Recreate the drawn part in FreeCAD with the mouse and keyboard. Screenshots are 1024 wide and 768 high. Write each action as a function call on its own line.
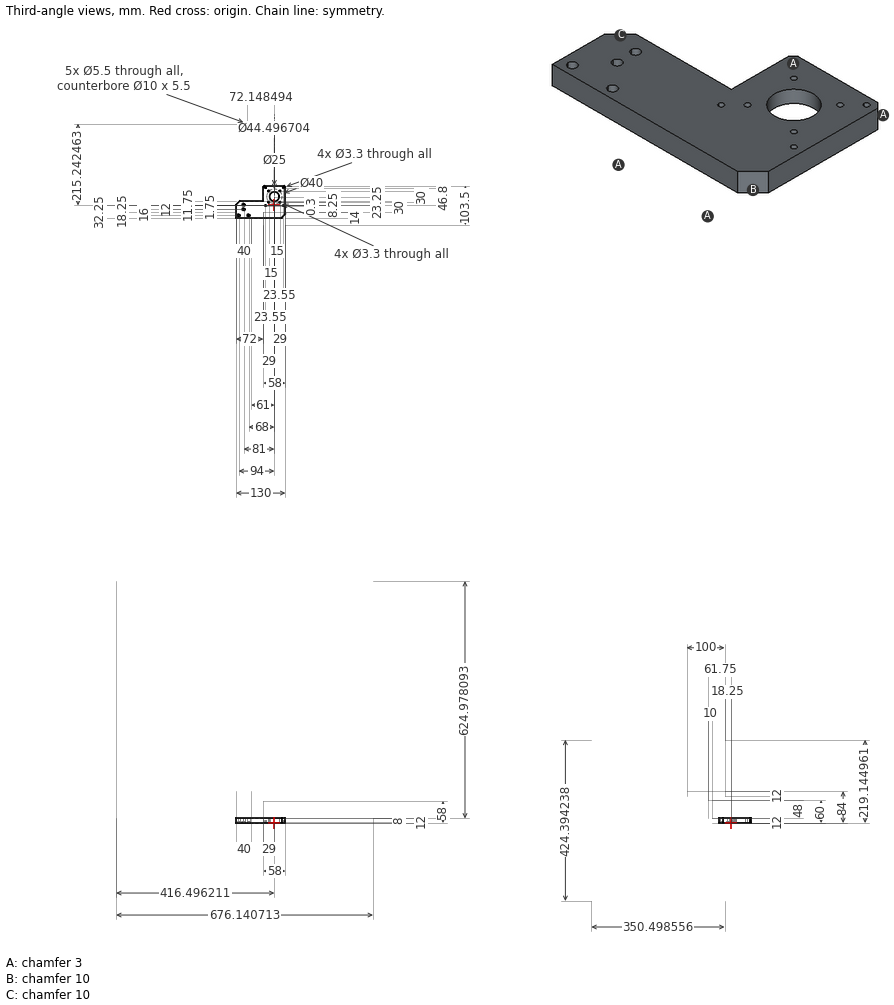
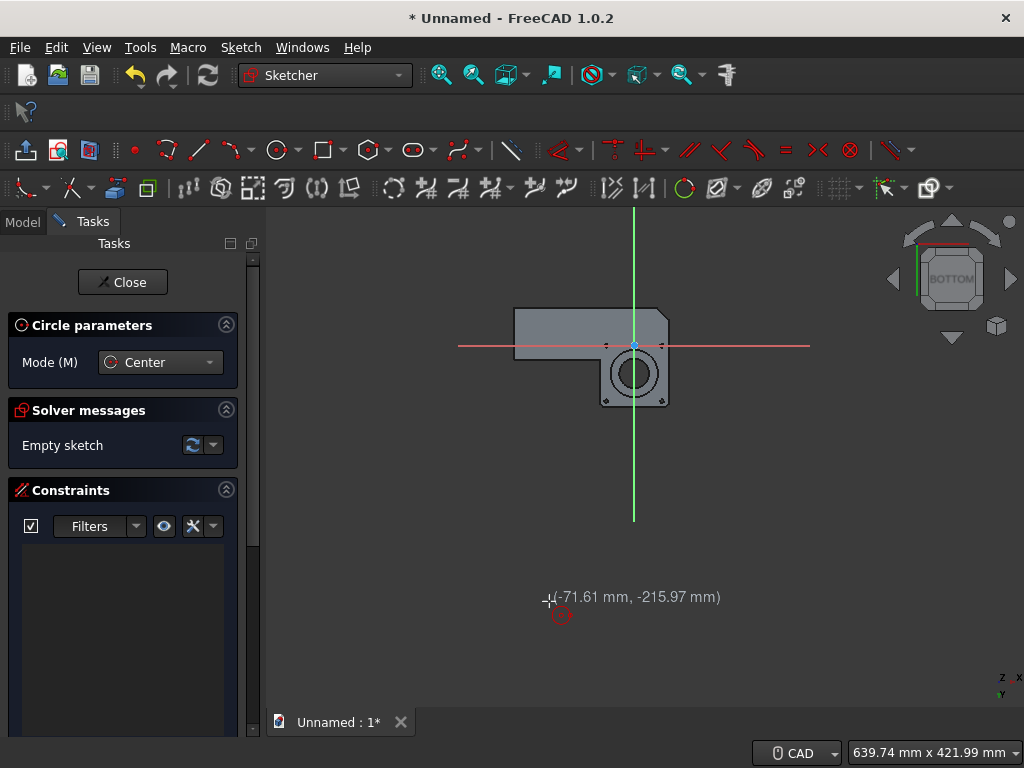
click(549, 601)
move(551, 599)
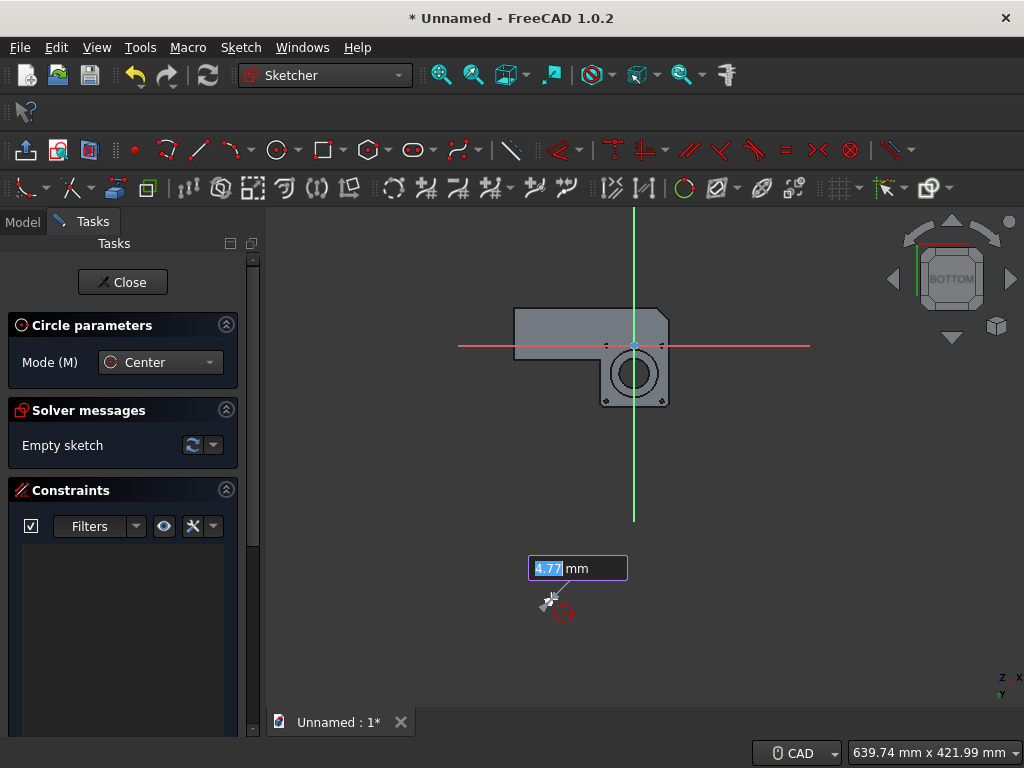
text(5.5)
key(Return)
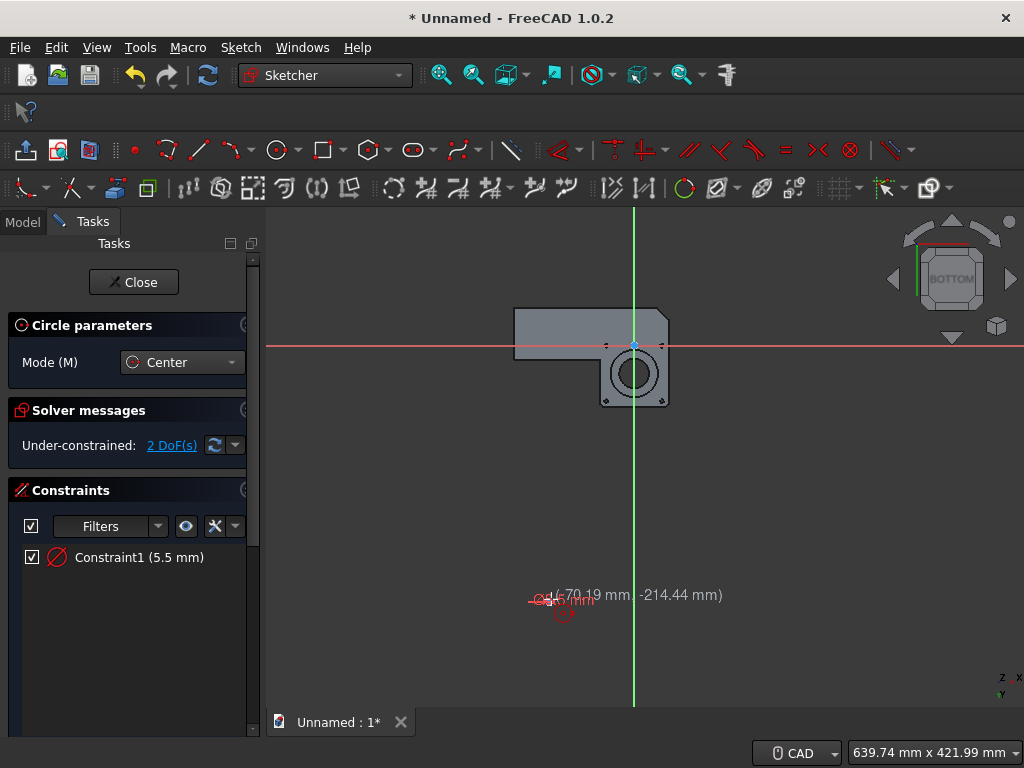
scroll(523, 315, up, 10)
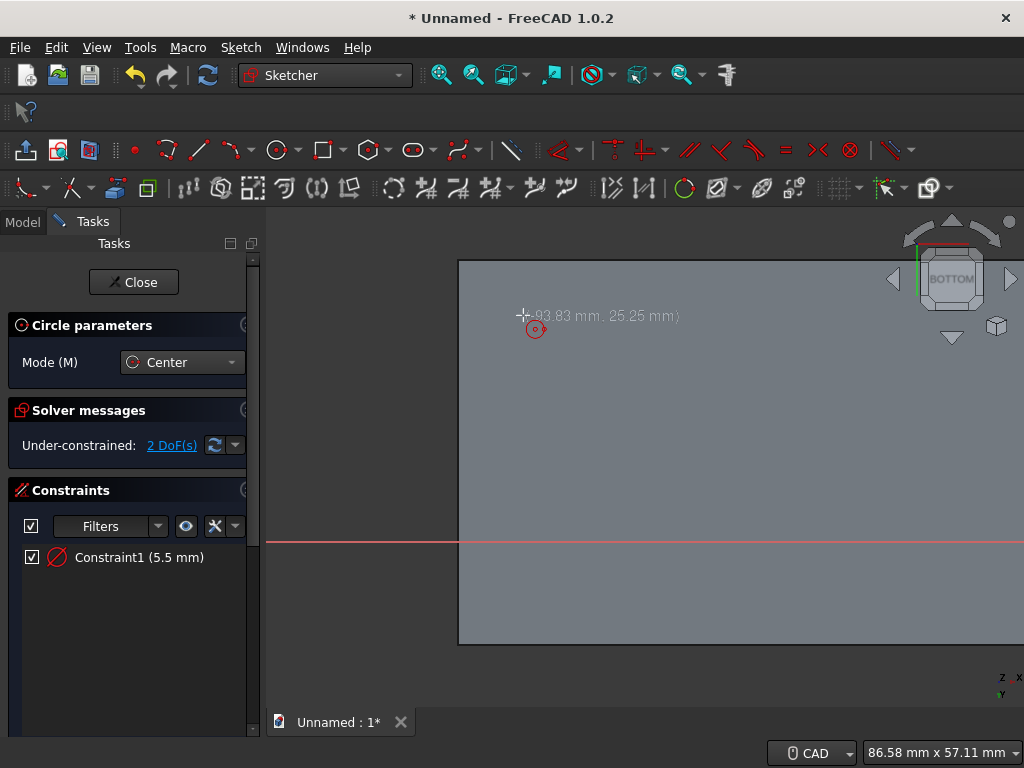
scroll(523, 314, down, 10)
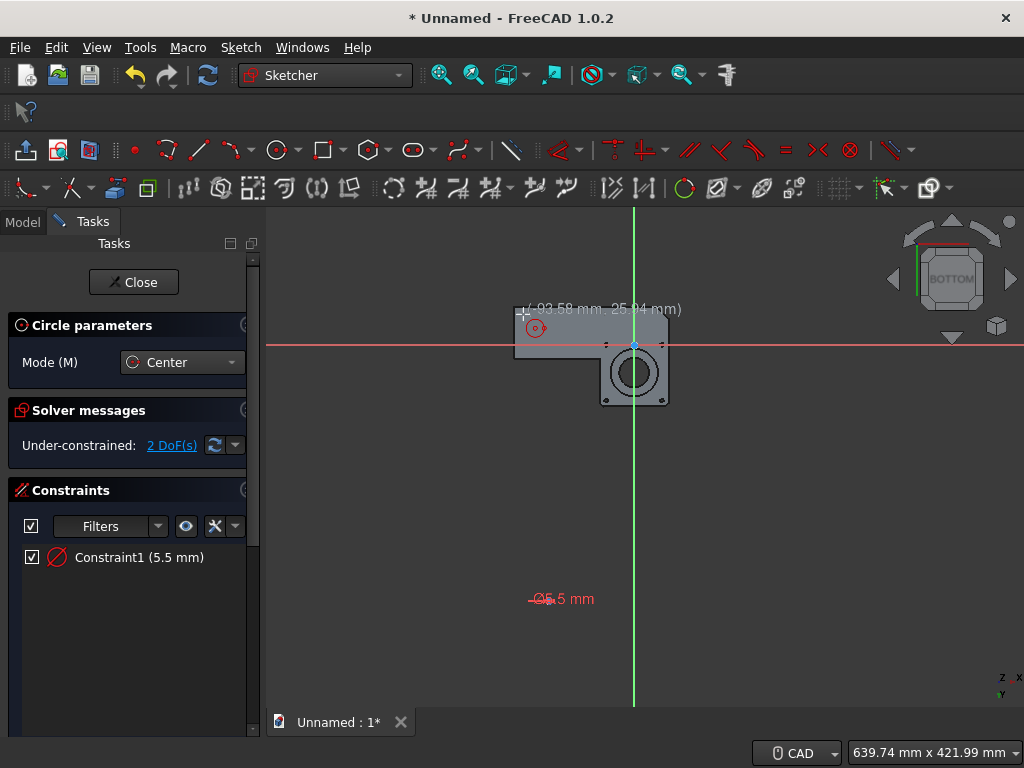
click(523, 314)
move(525, 312)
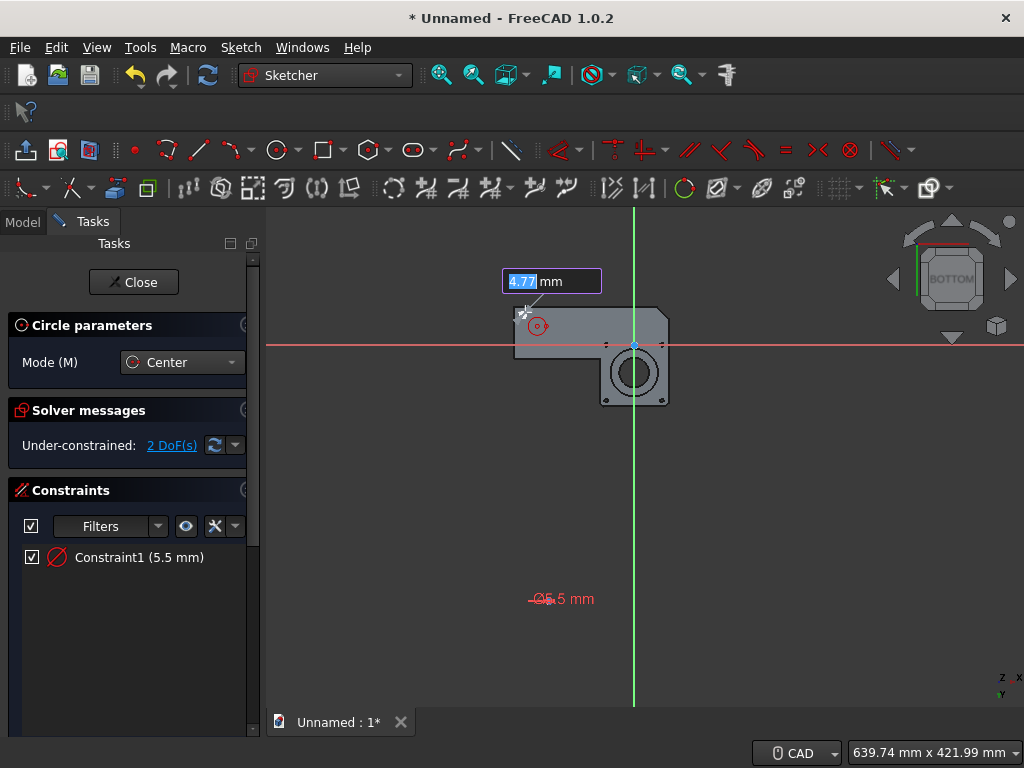
text(5.5)
key(Return)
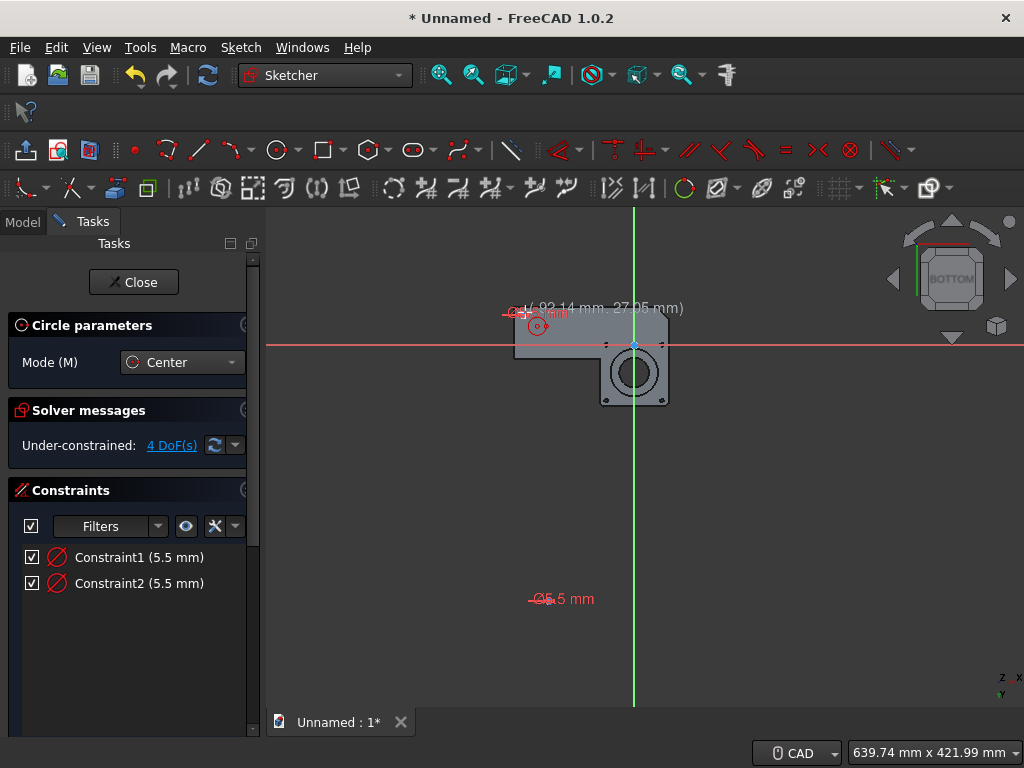
scroll(554, 314, up, 10)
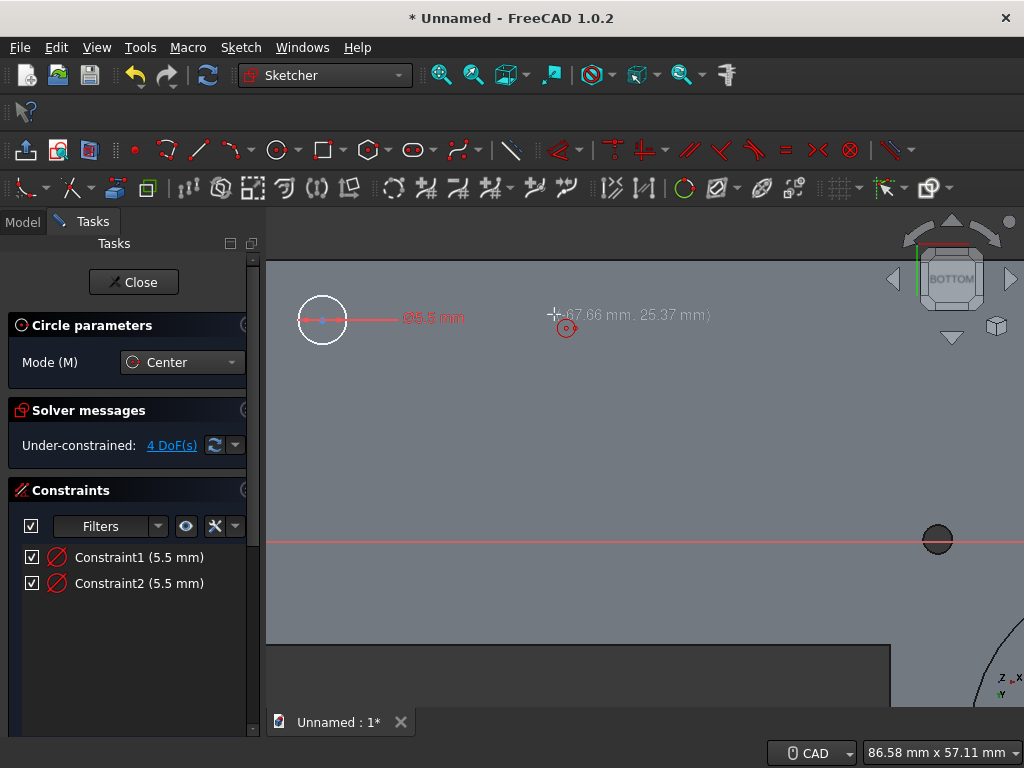
scroll(554, 314, down, 10)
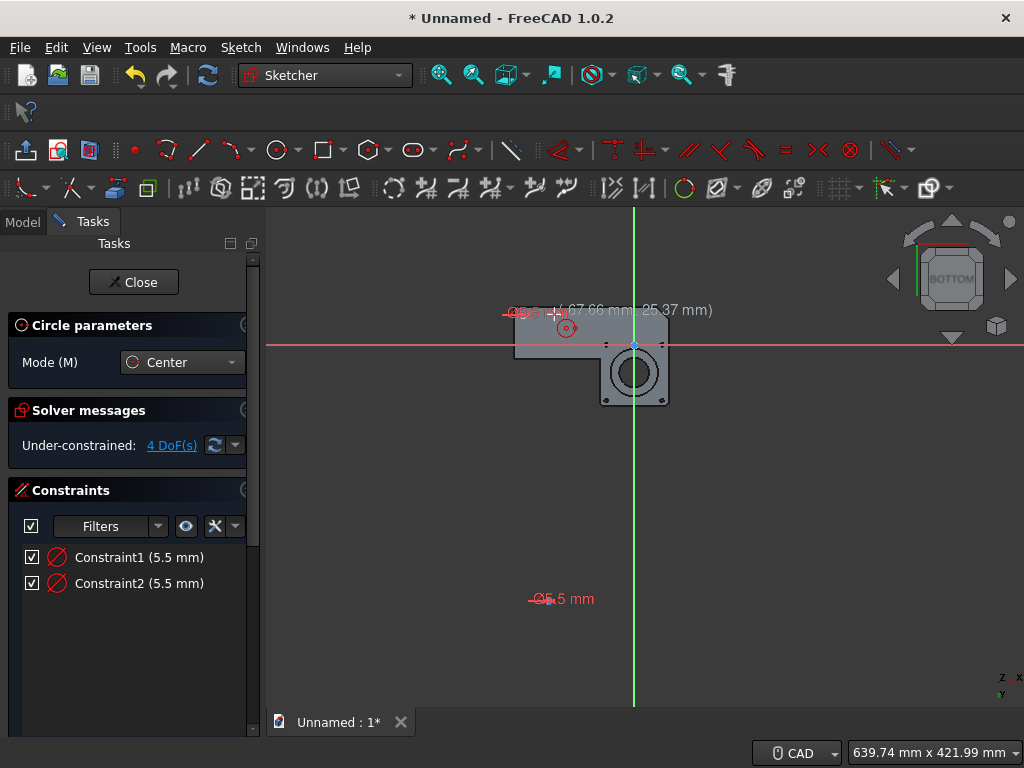
click(554, 314)
move(556, 312)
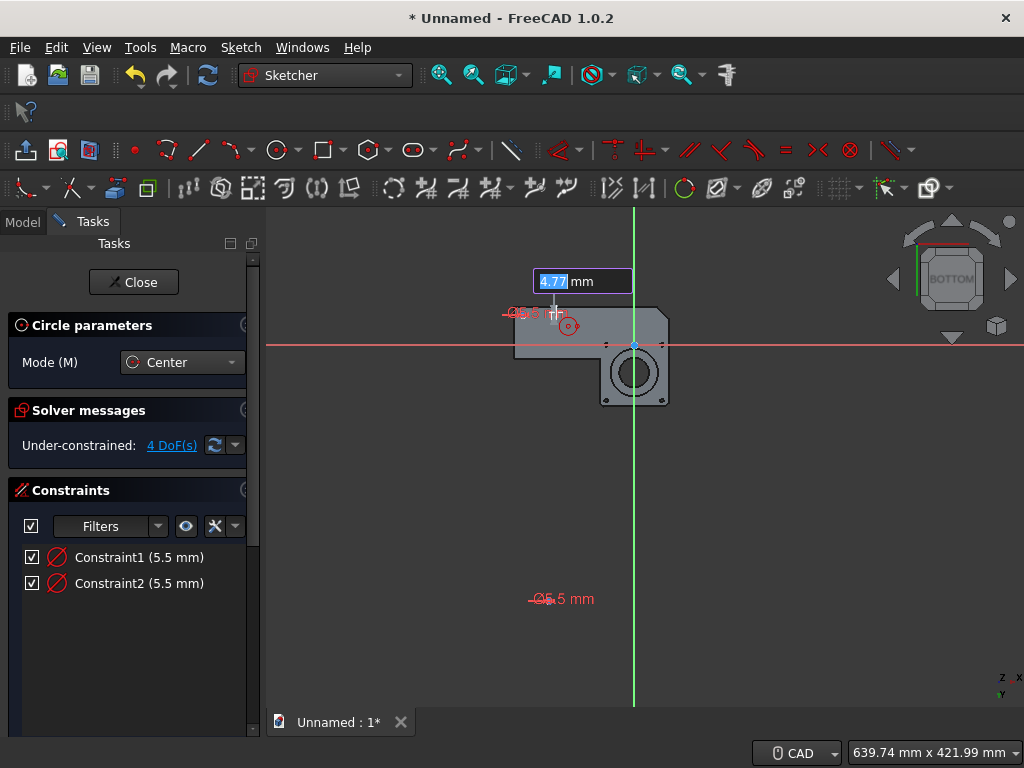
text(5.5)
key(Return)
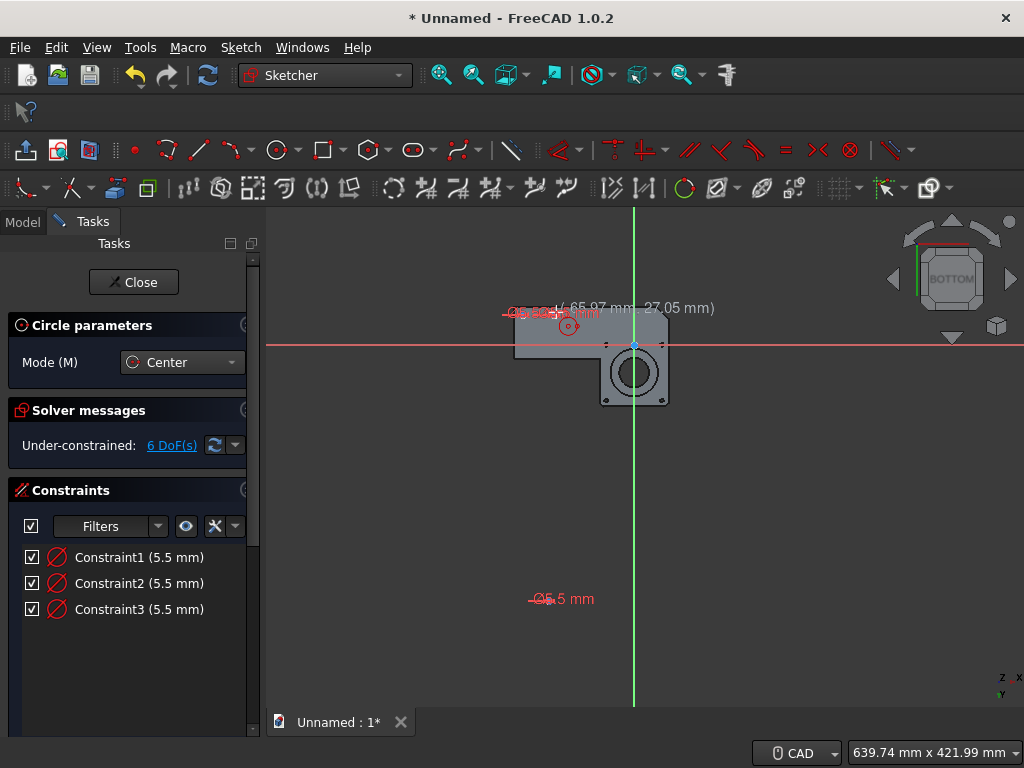
scroll(538, 333, up, 10)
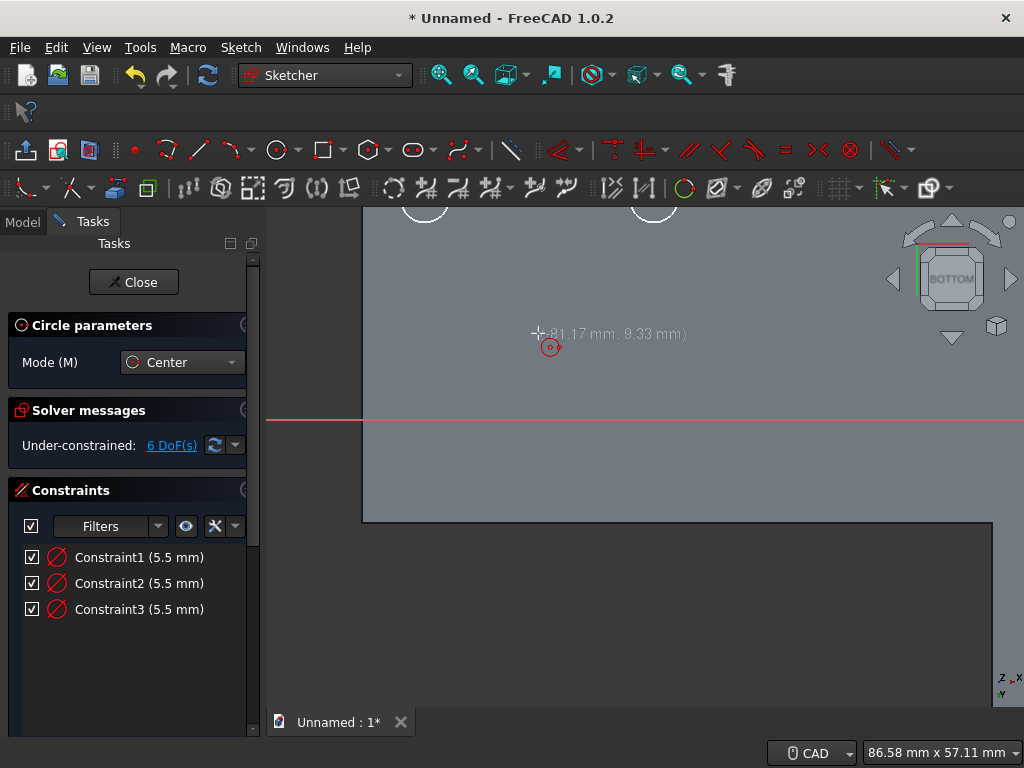
scroll(538, 333, down, 10)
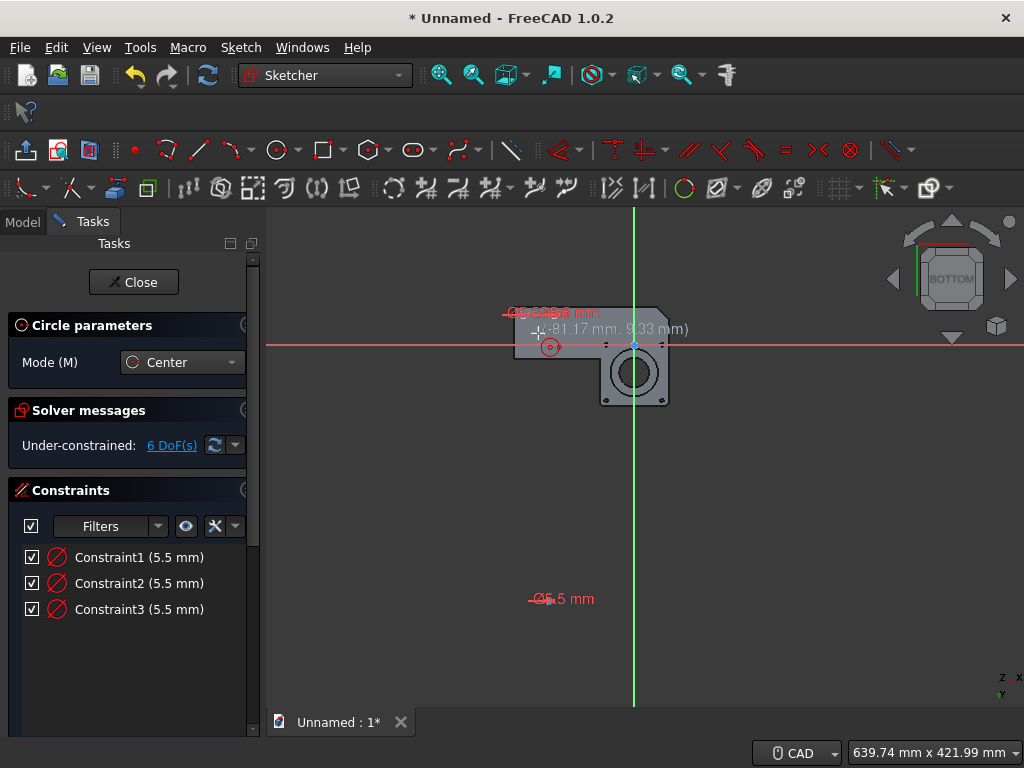
scroll(538, 333, up, 2)